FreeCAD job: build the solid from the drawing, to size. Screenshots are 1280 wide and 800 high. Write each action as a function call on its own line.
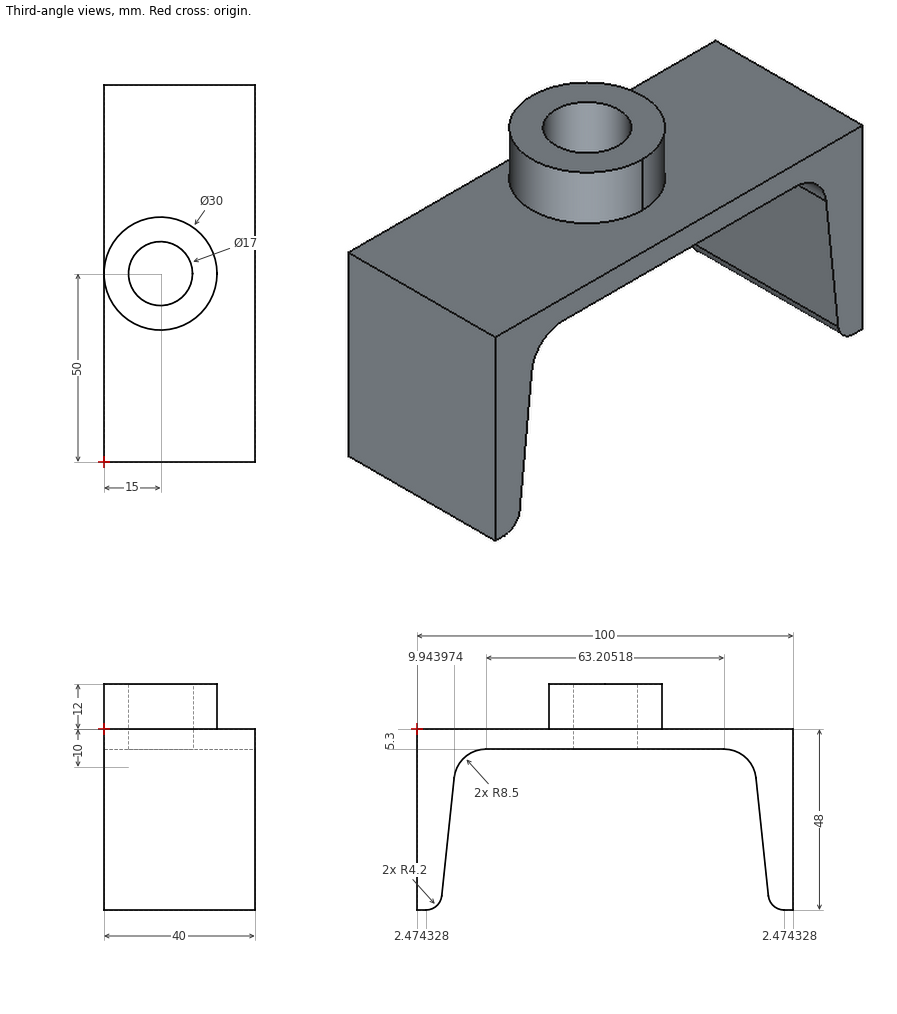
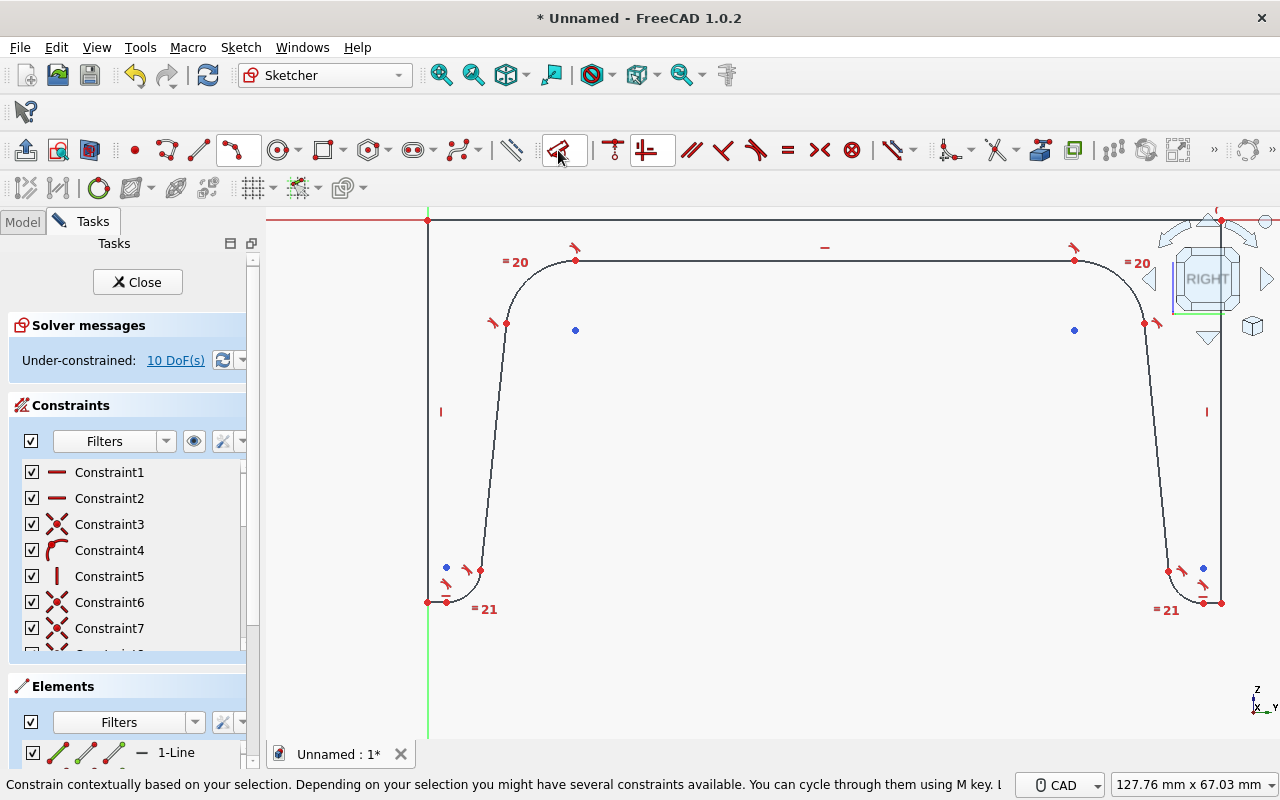
click(546, 267)
click(532, 238)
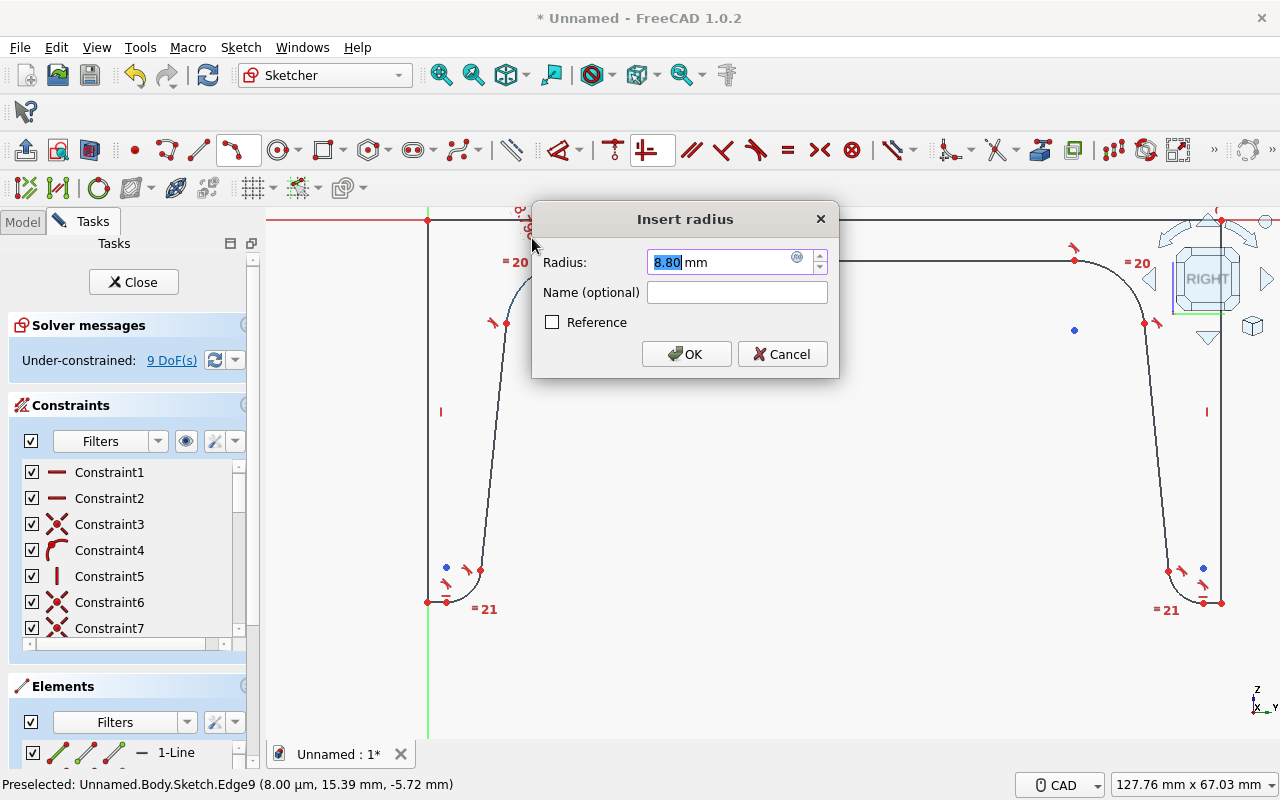
text(8.5)
key(Return)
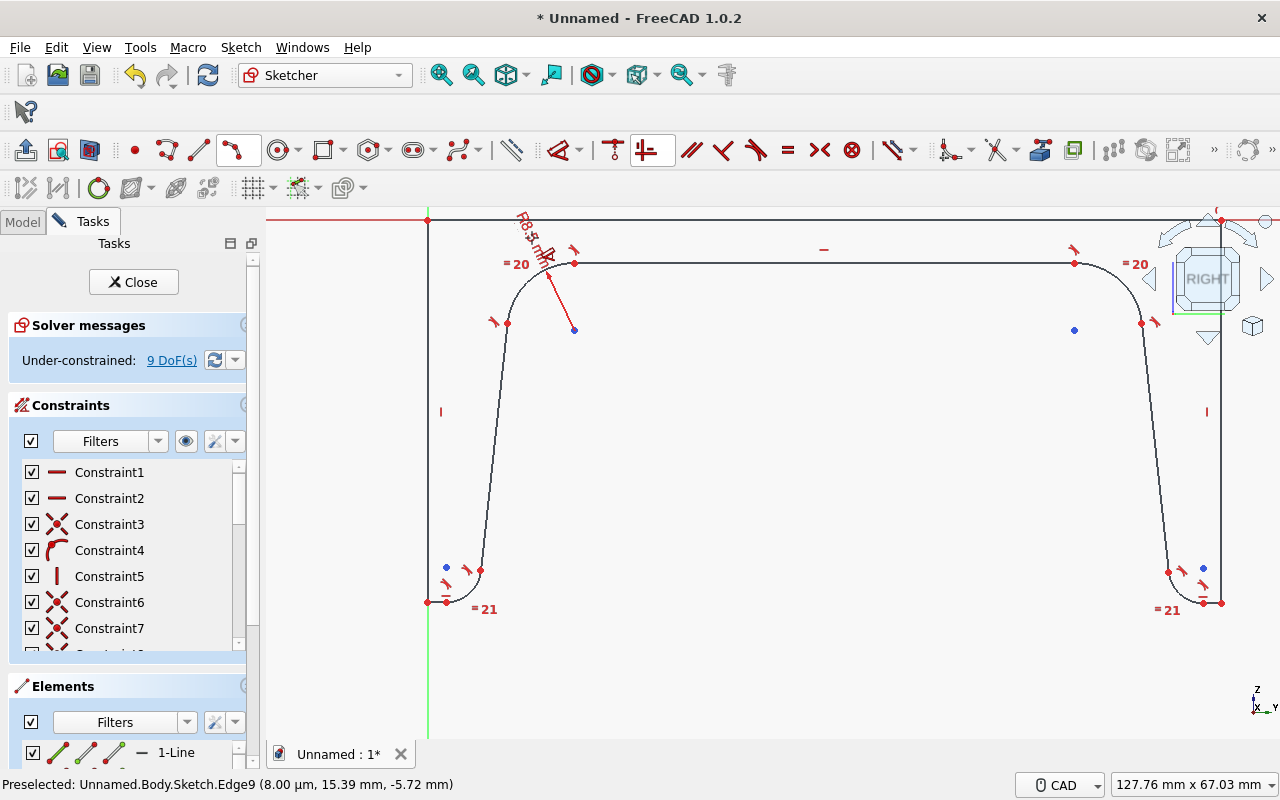
scroll(460, 599, down, 2)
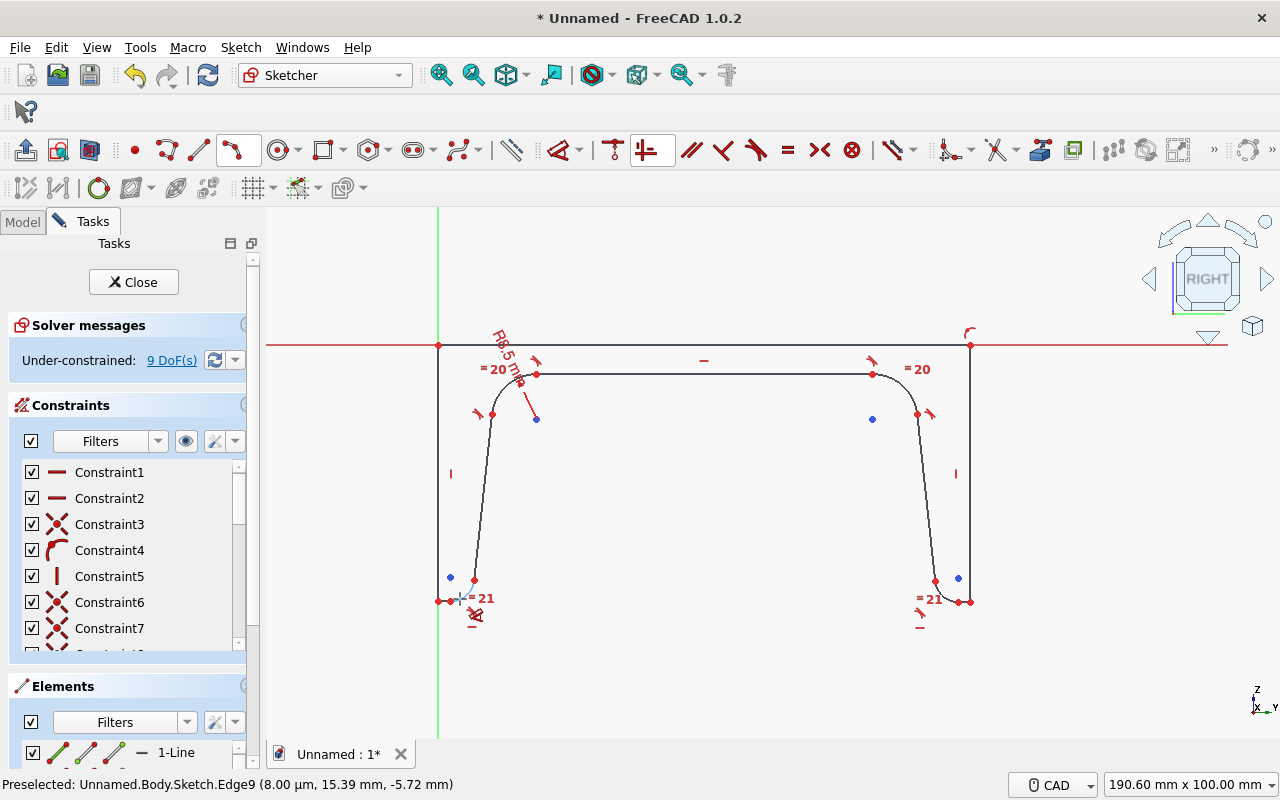
scroll(939, 591, up, 3)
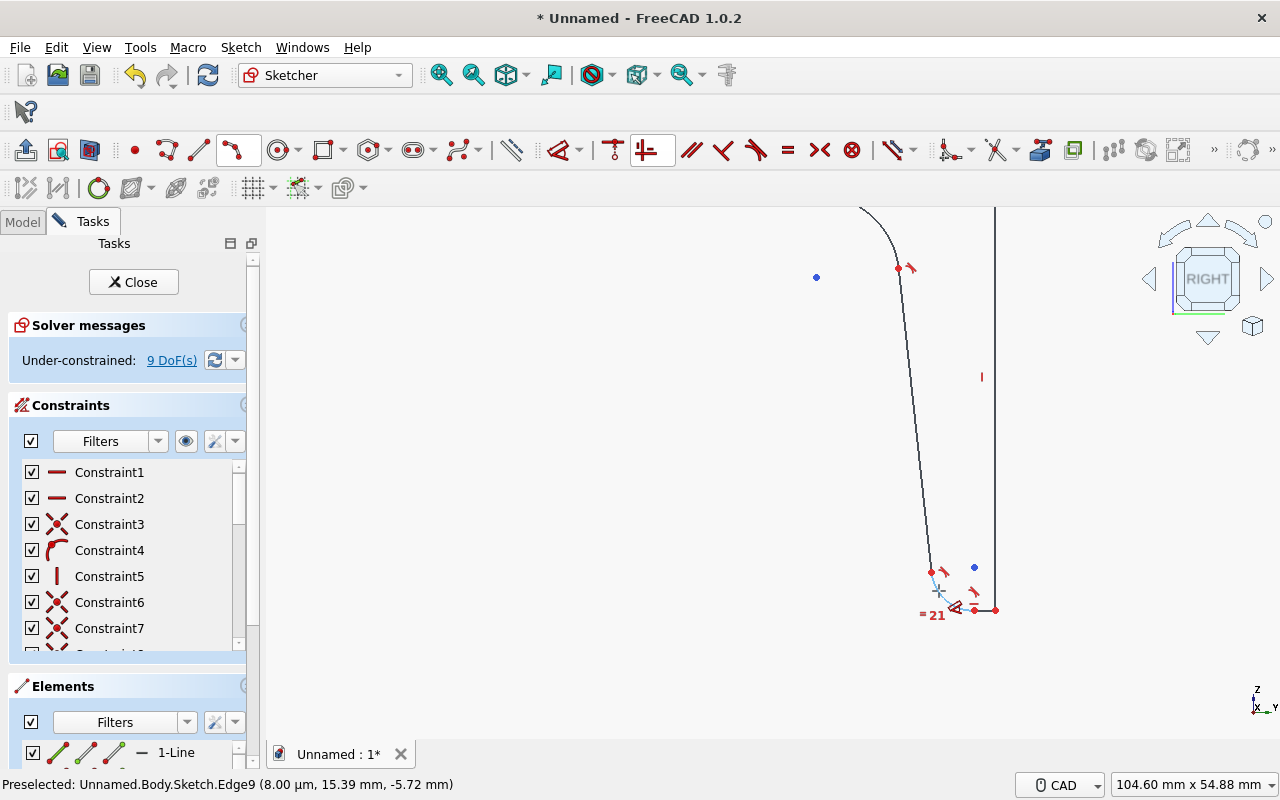
click(938, 590)
click(911, 607)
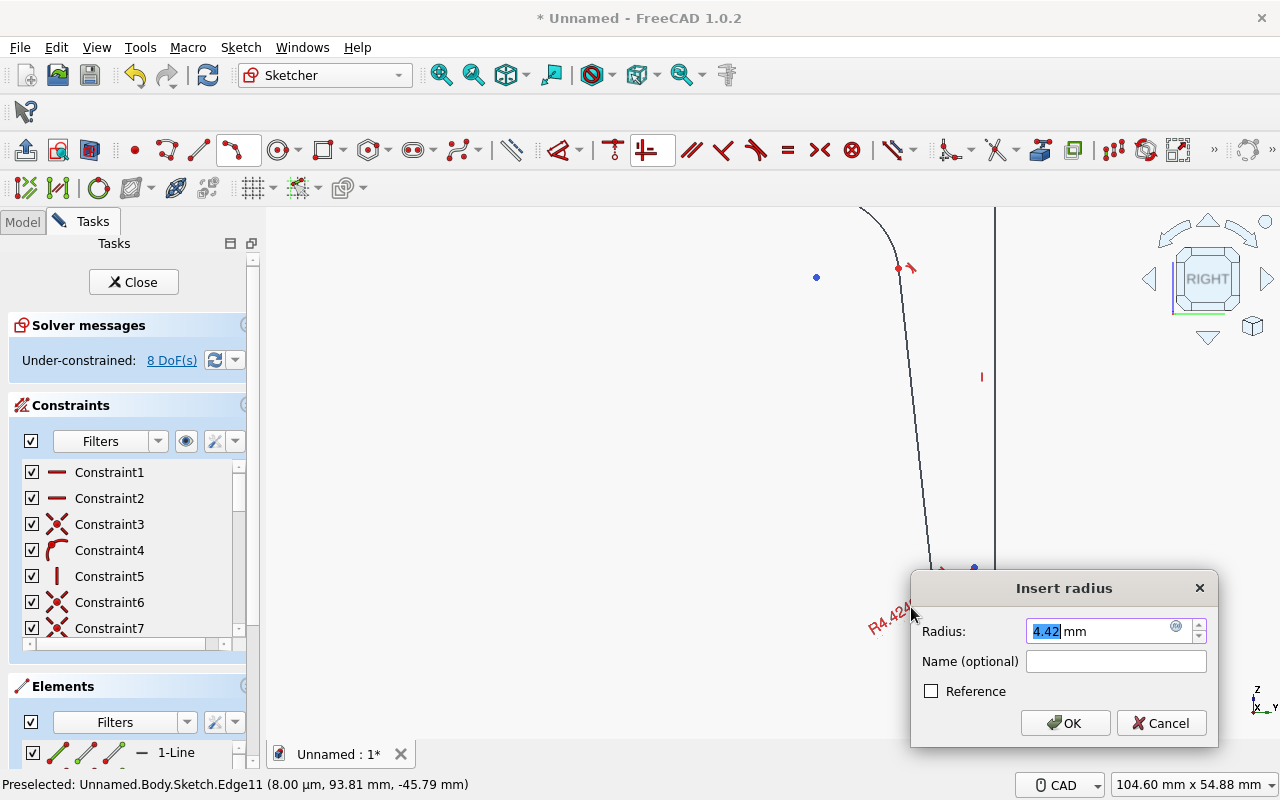
text(4.2)
key(Return)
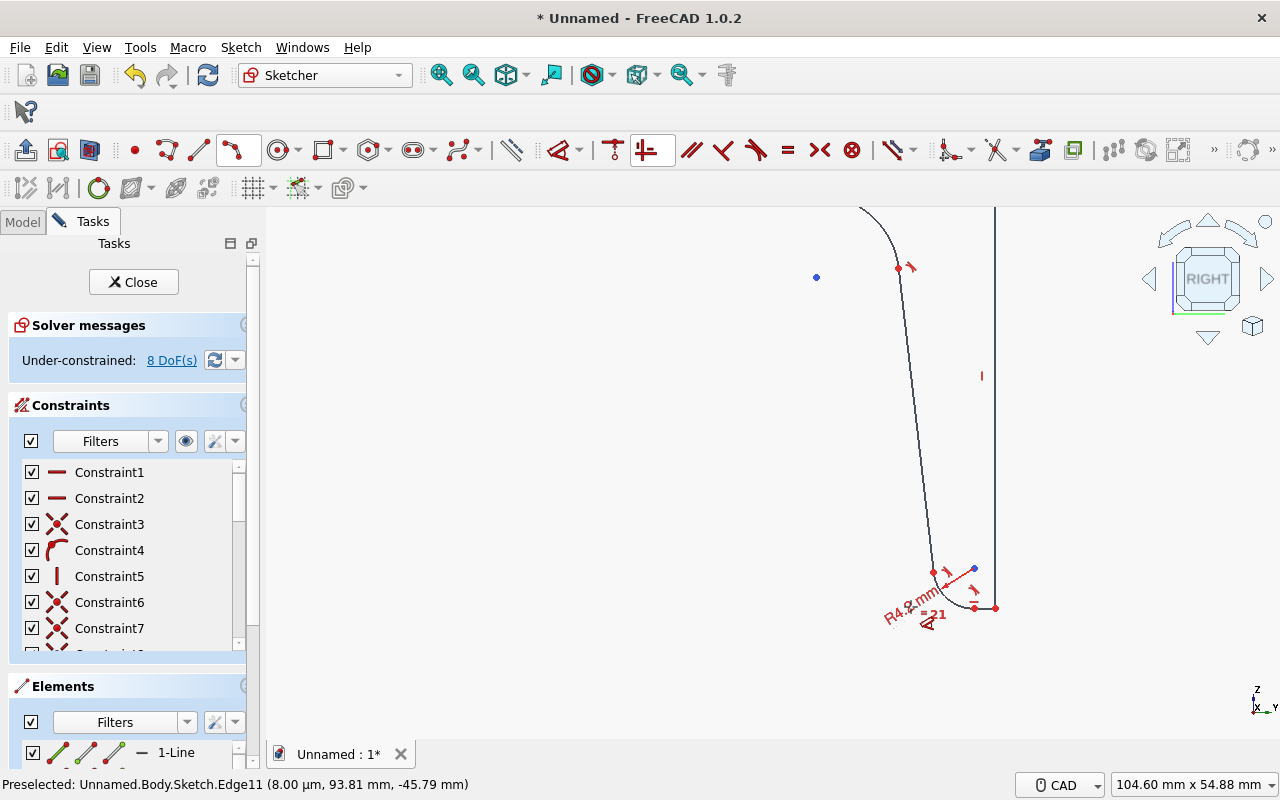
click(995, 469)
click(1029, 422)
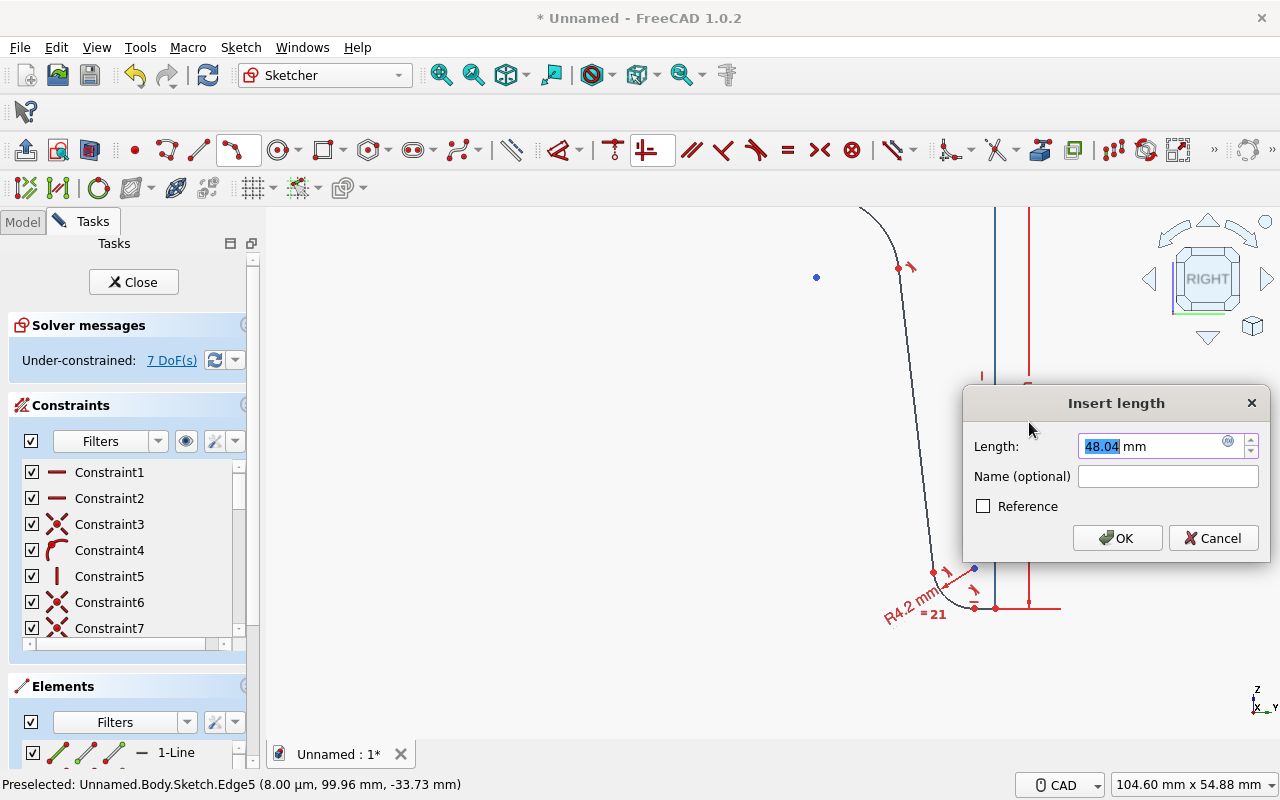
text(48)
key(Return)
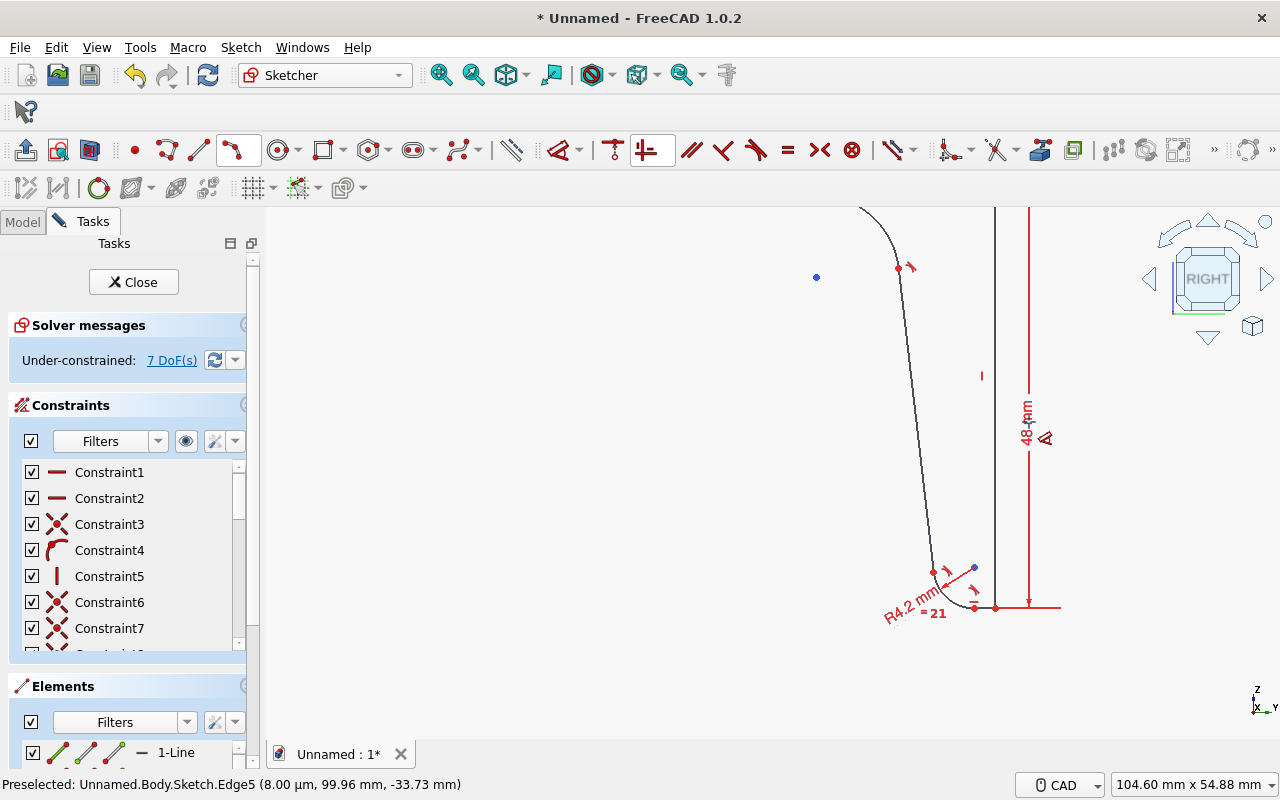
scroll(940, 591, down, 3)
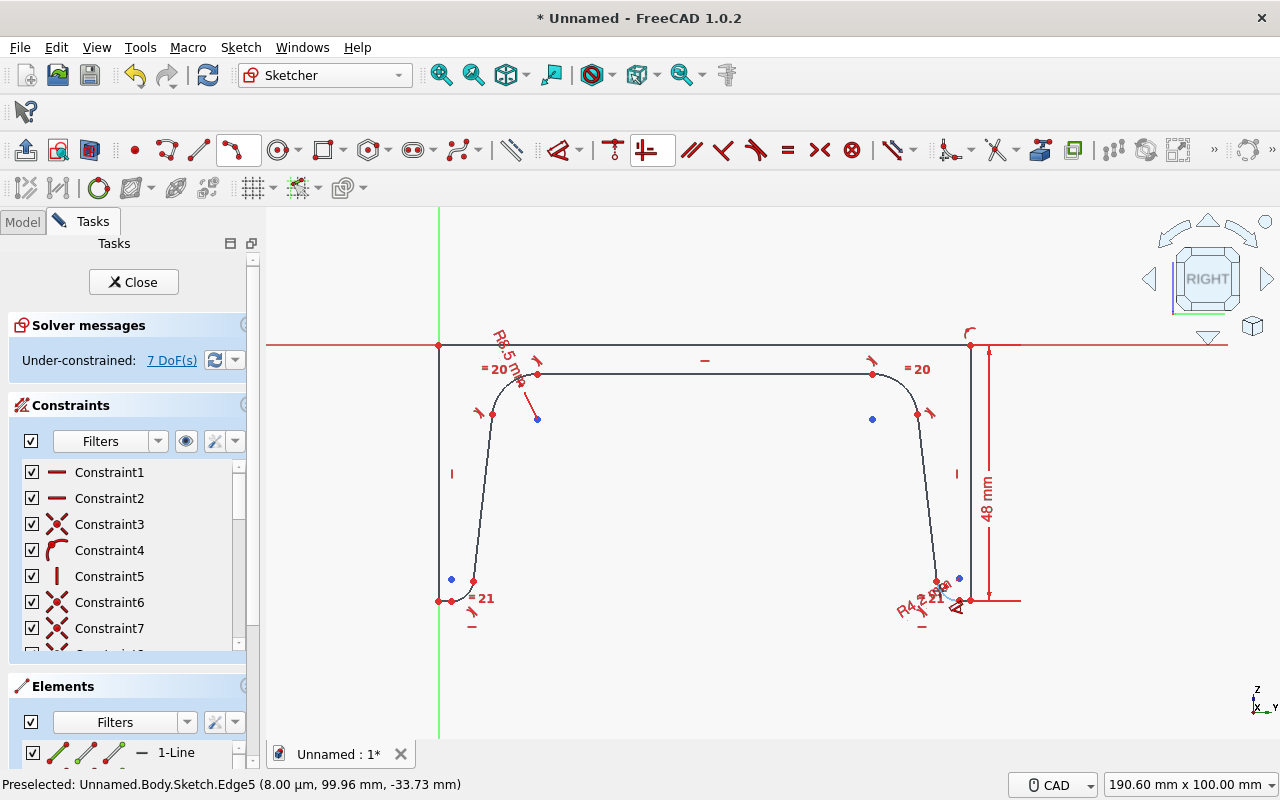
click(439, 422)
click(405, 473)